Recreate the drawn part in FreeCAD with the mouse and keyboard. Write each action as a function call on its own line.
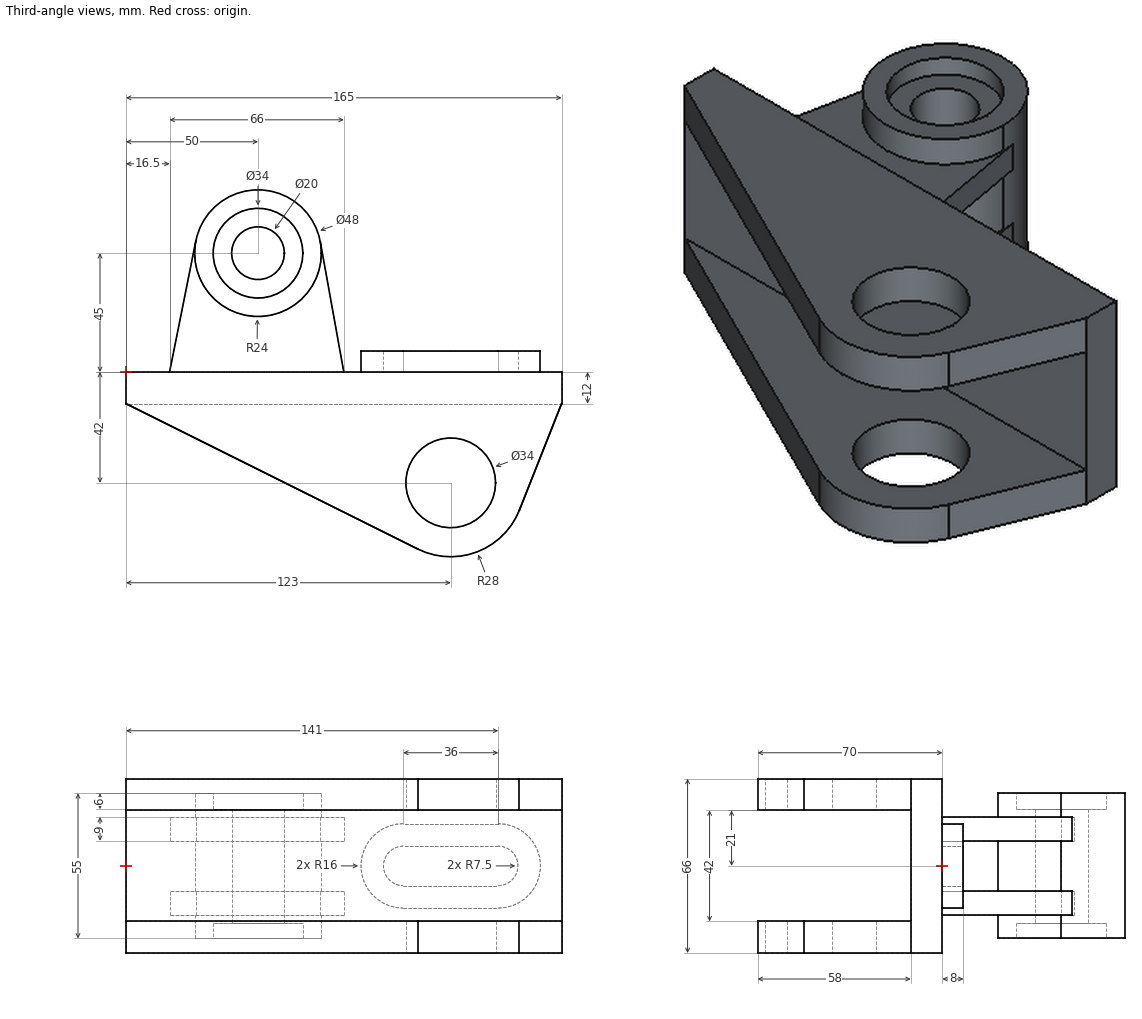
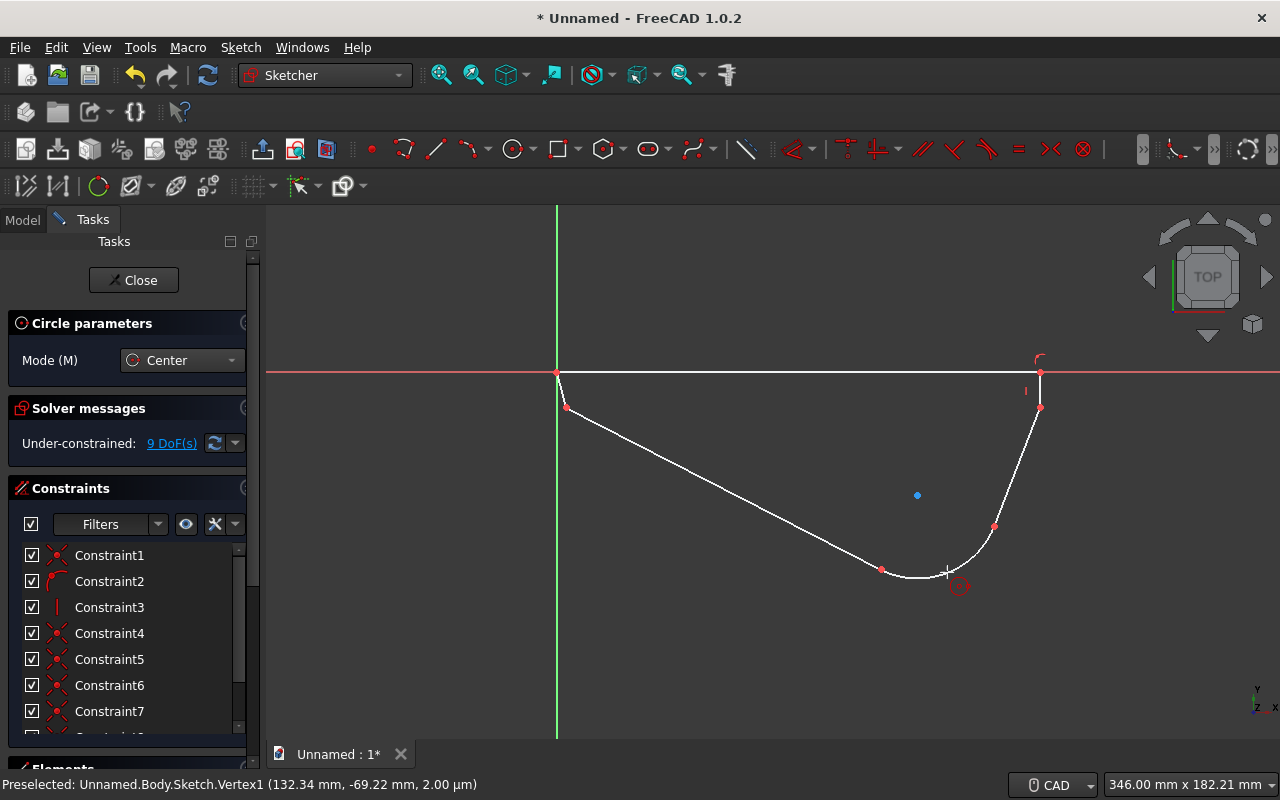
click(917, 495)
move(953, 460)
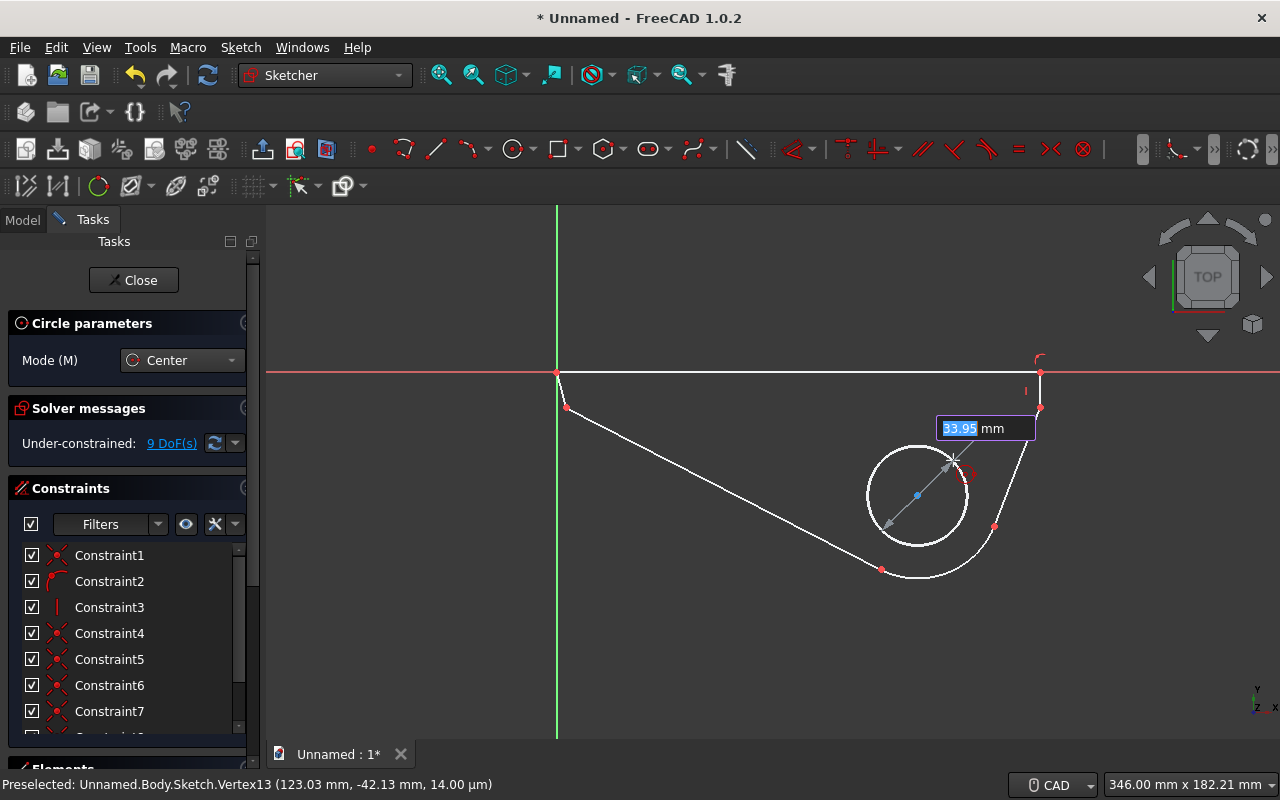
text(34)
key(Return)
key(Escape)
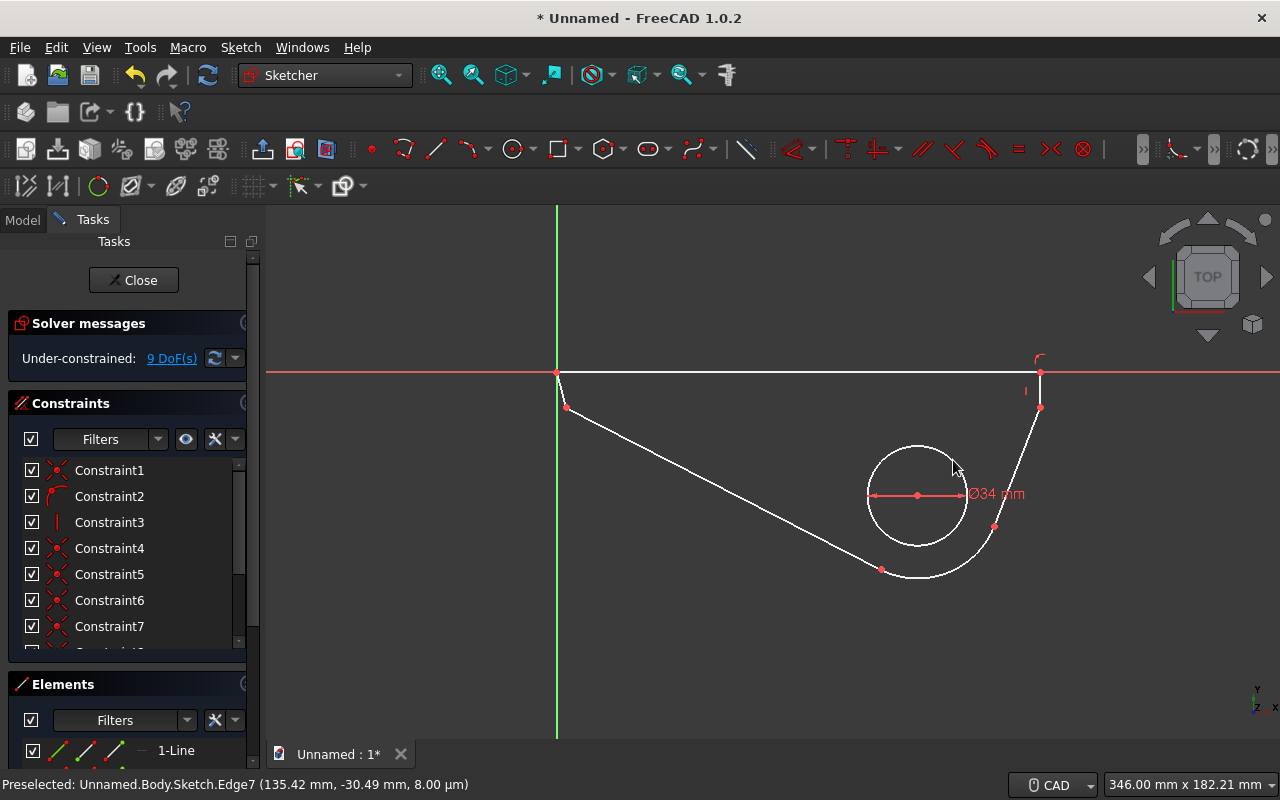
click(1026, 444)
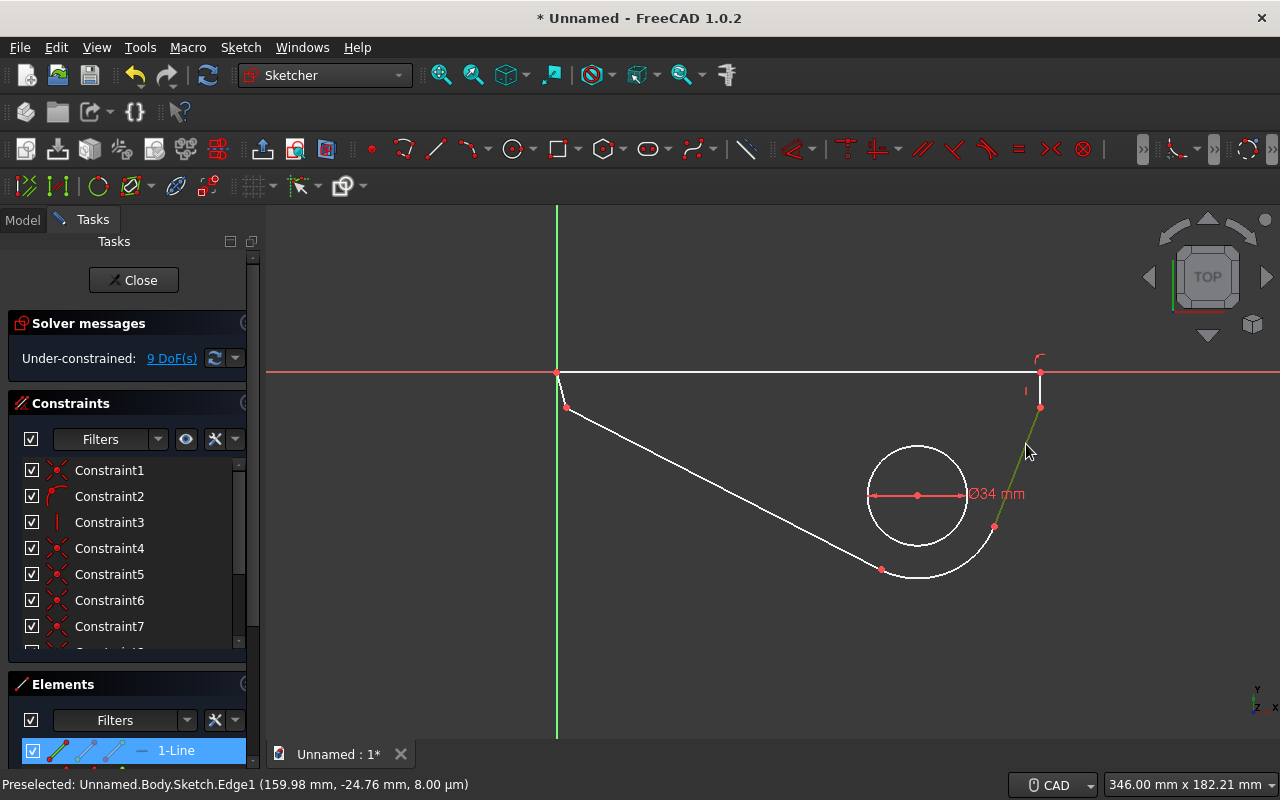
click(920, 578)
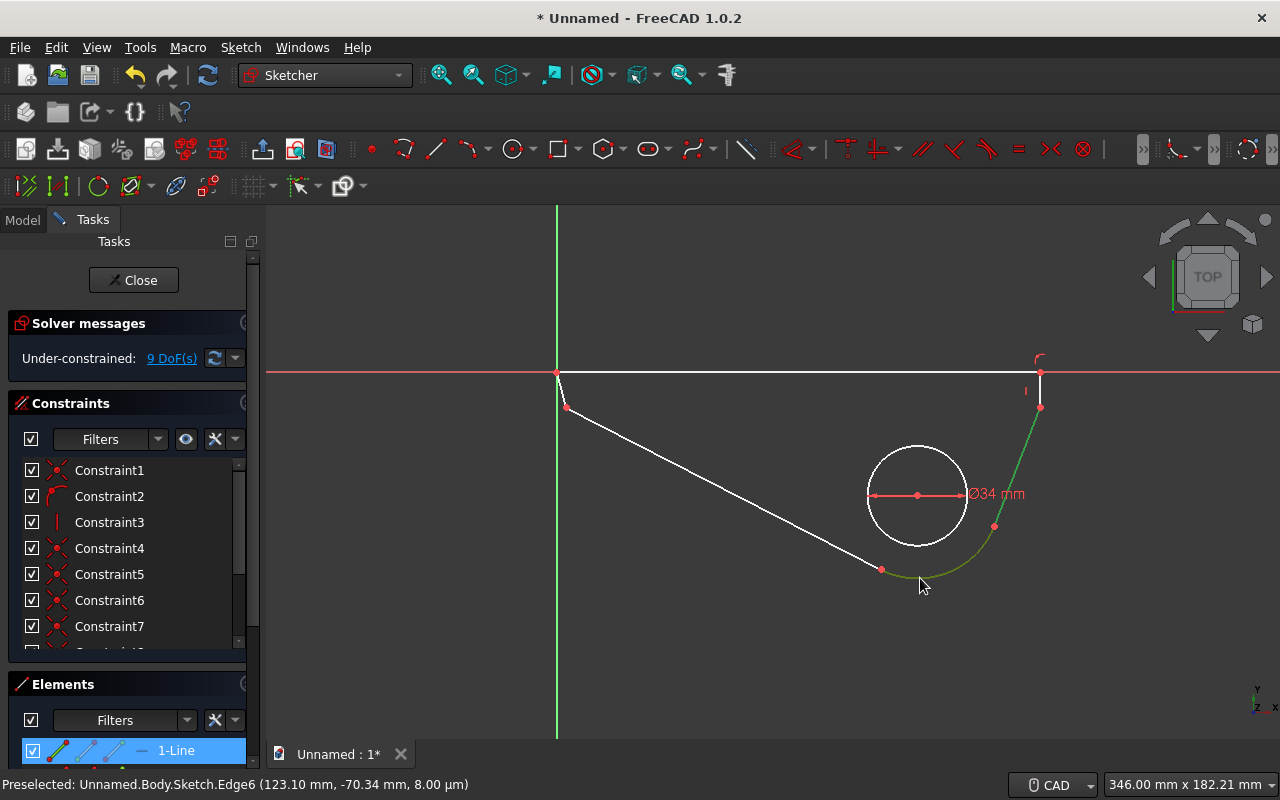
key(t)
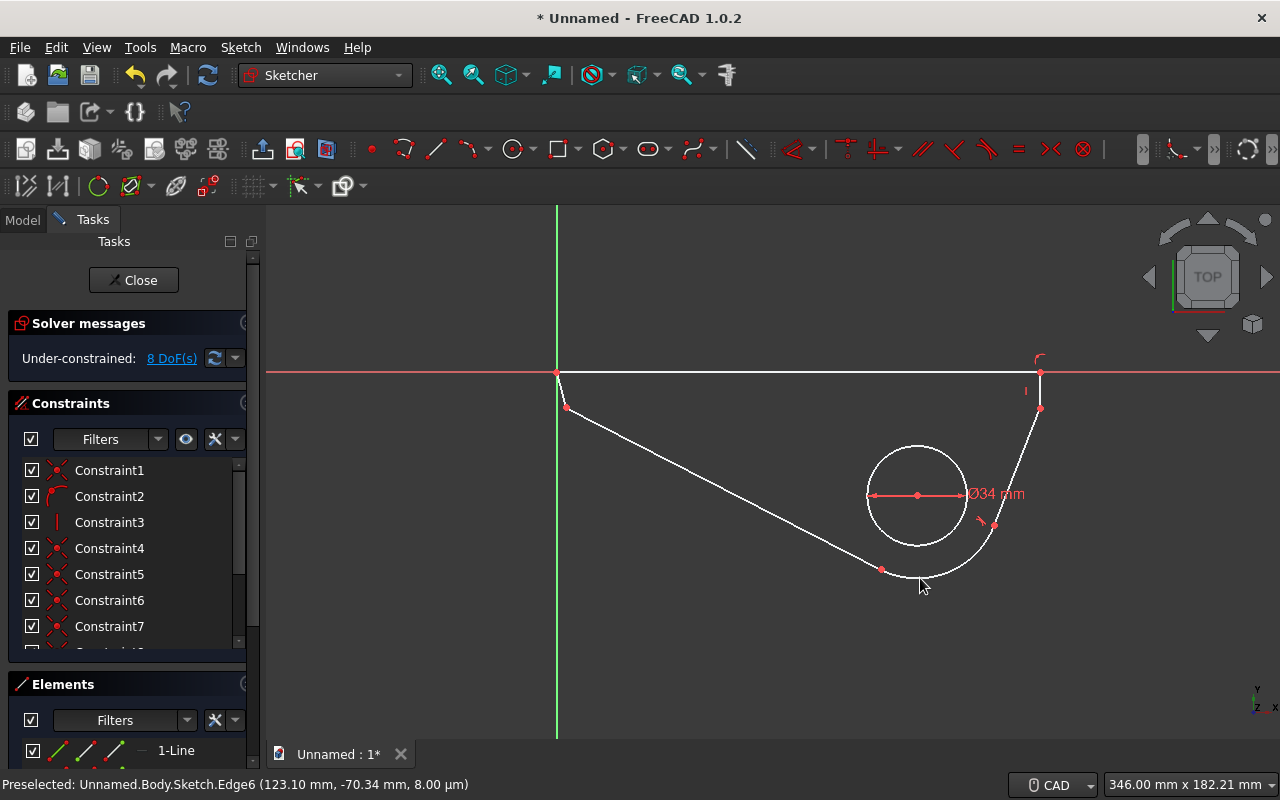
click(660, 457)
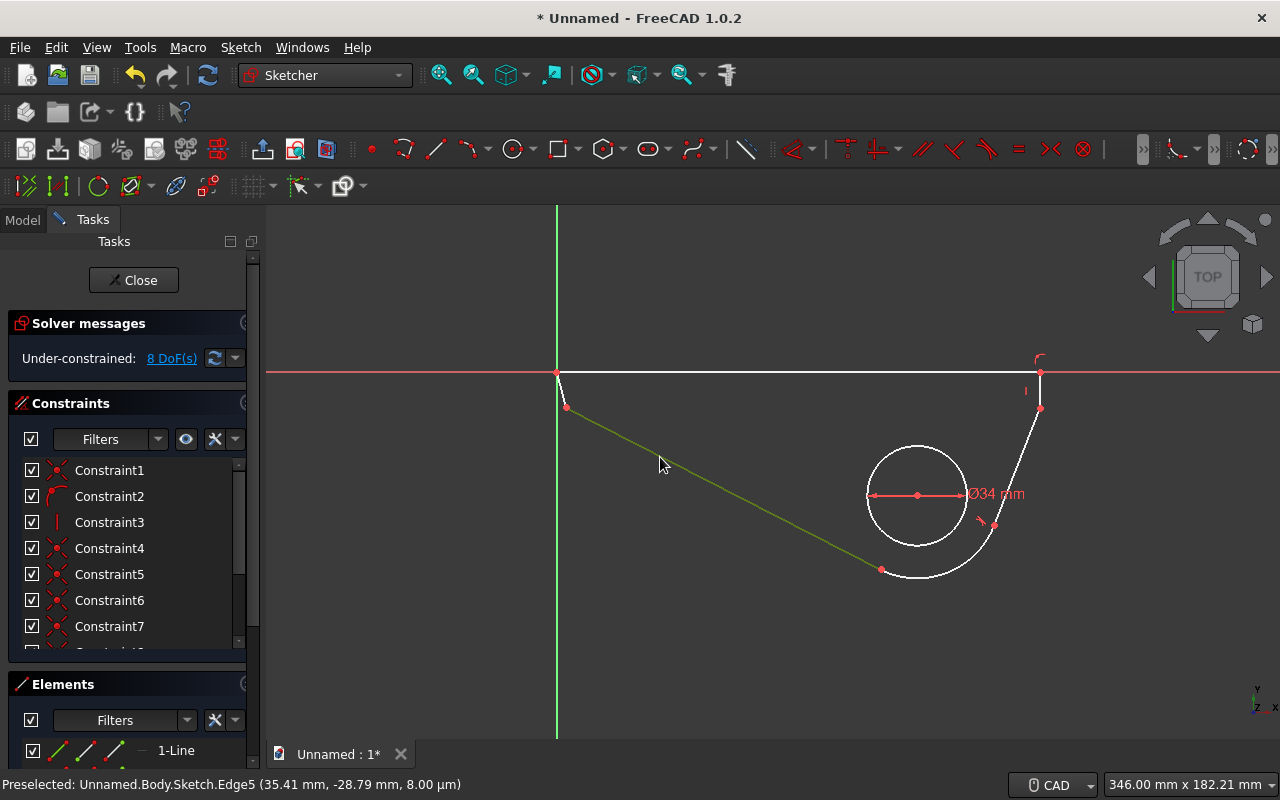
click(921, 578)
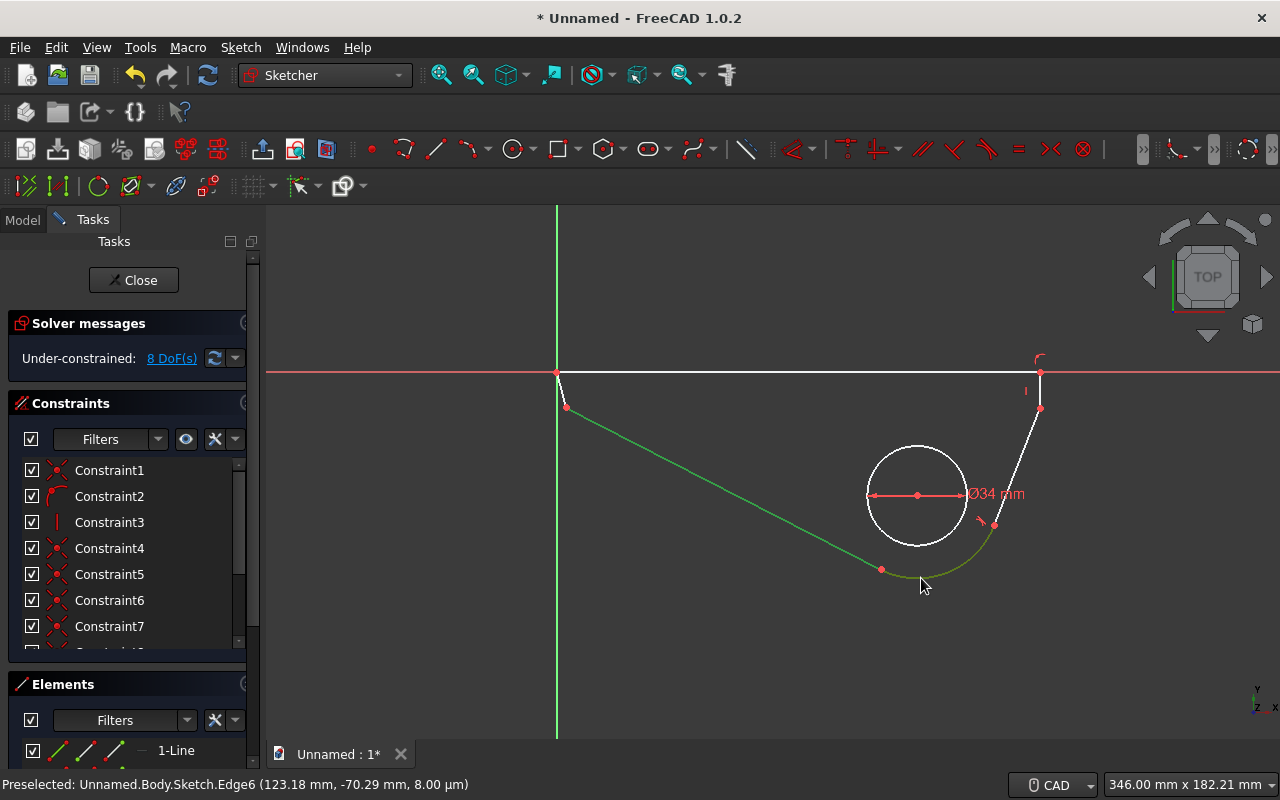
click(988, 150)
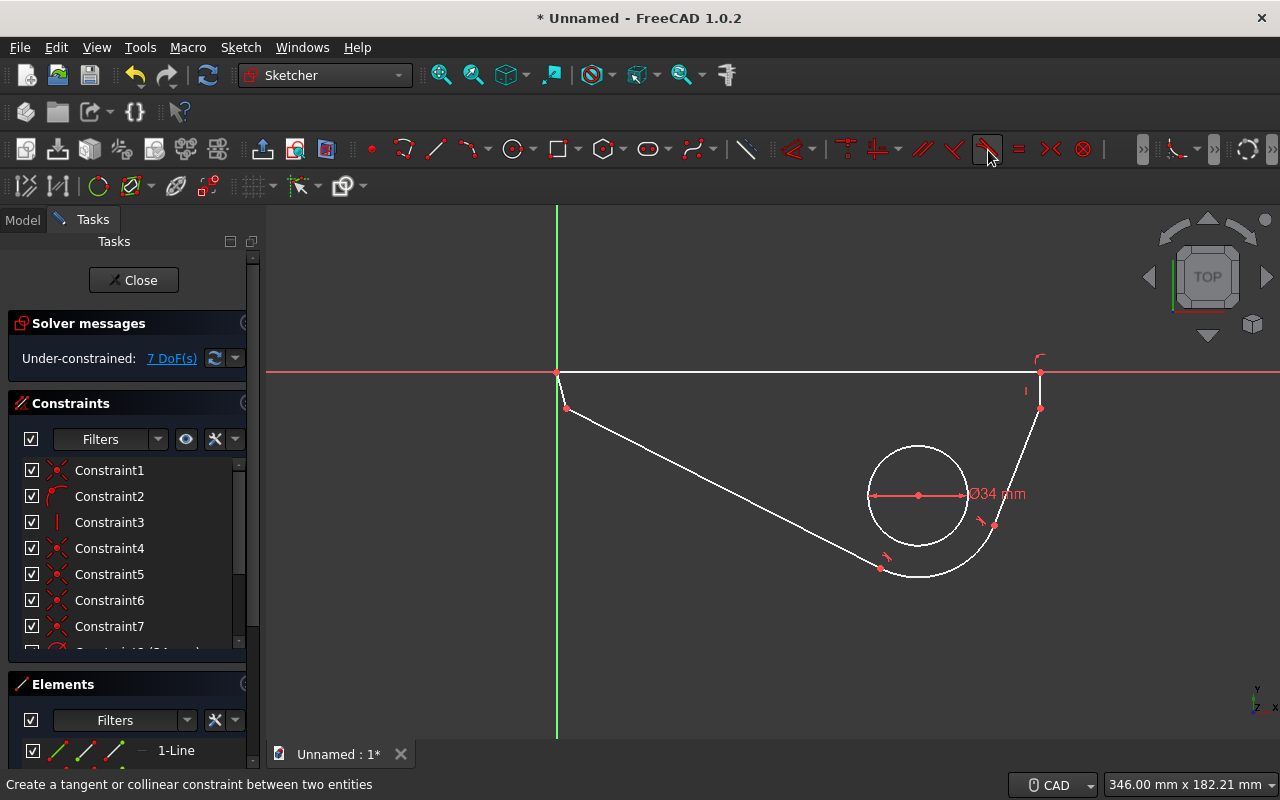
scroll(560, 383, up, 2)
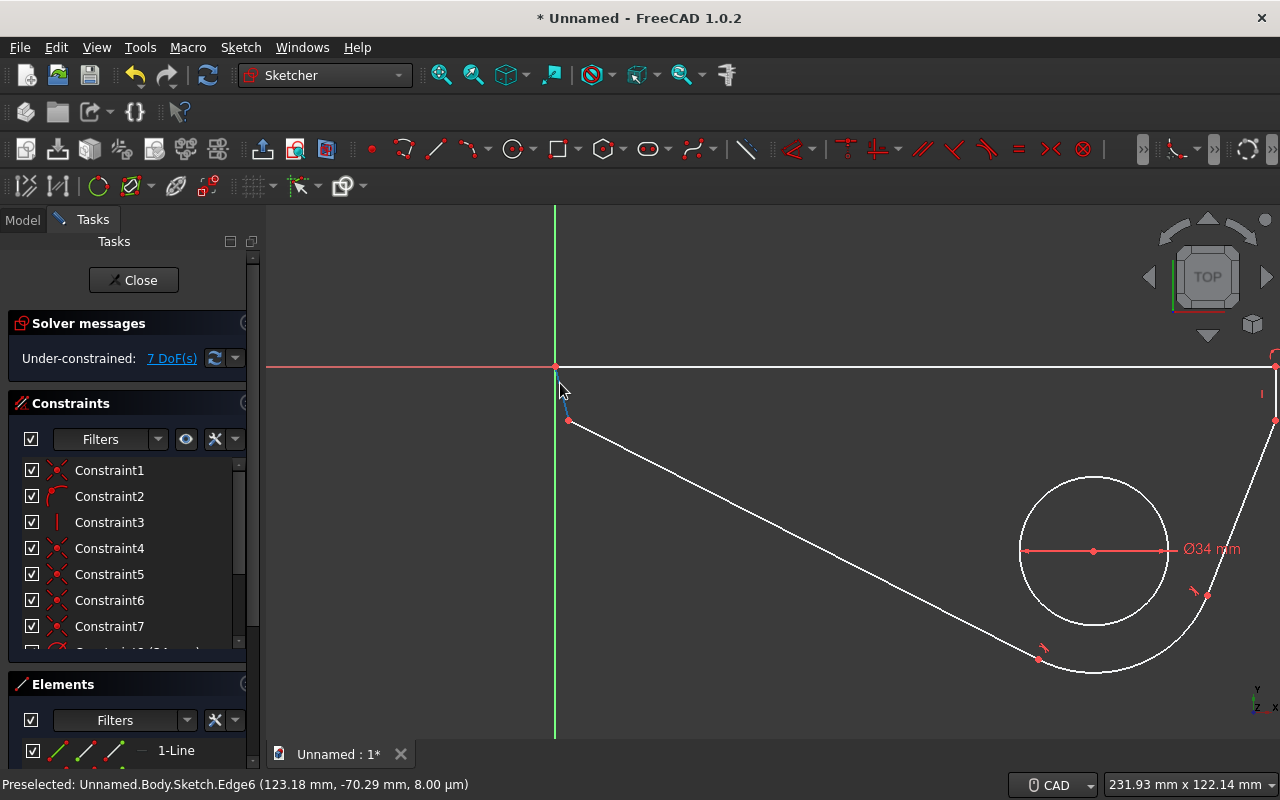
click(559, 383)